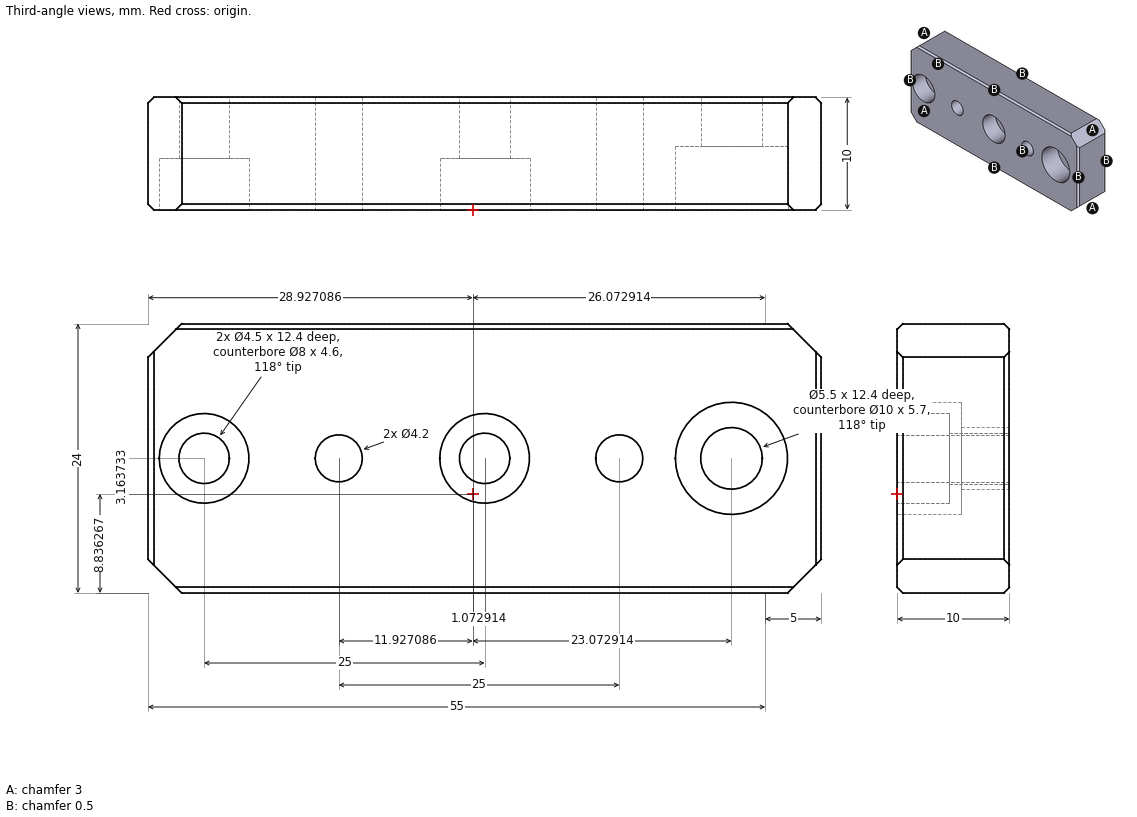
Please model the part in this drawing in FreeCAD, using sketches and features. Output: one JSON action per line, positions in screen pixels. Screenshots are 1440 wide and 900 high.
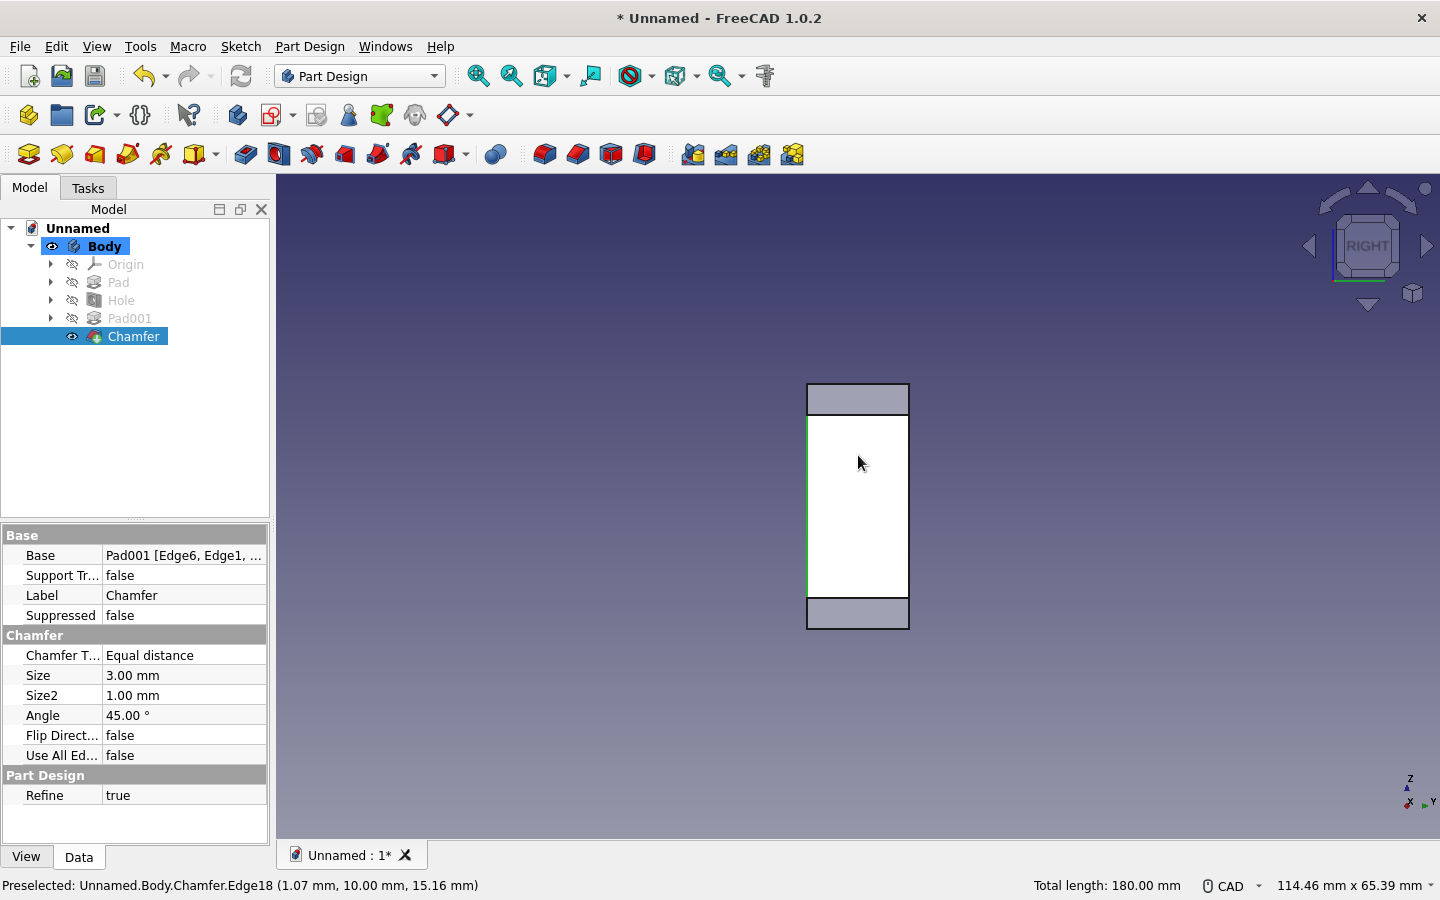
{"action": "left_click", "coordinate": [909, 505], "text": "ctrl"}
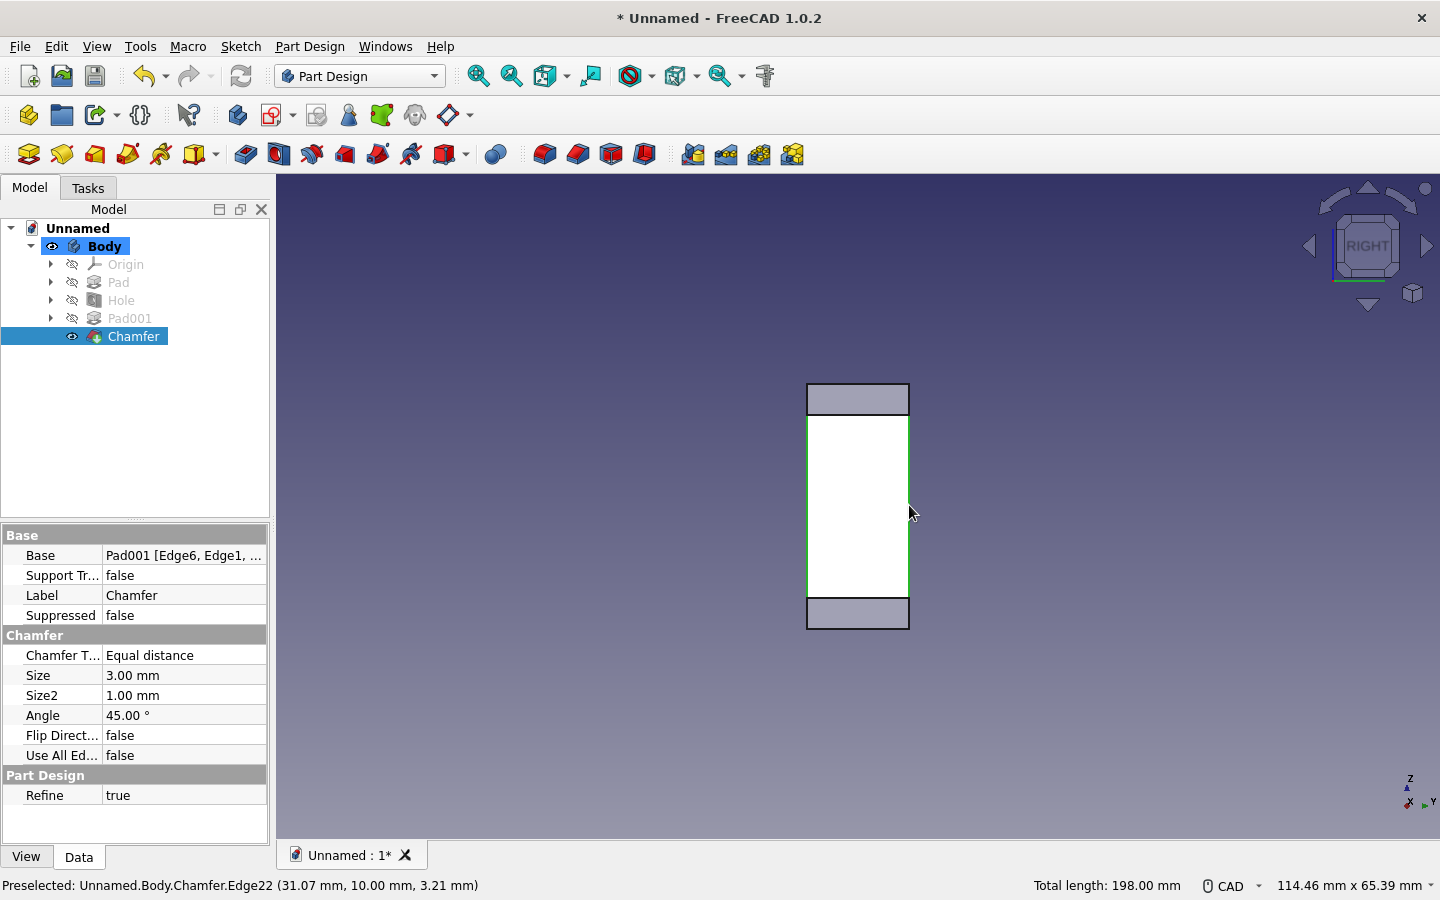
{"action": "key", "text": "5"}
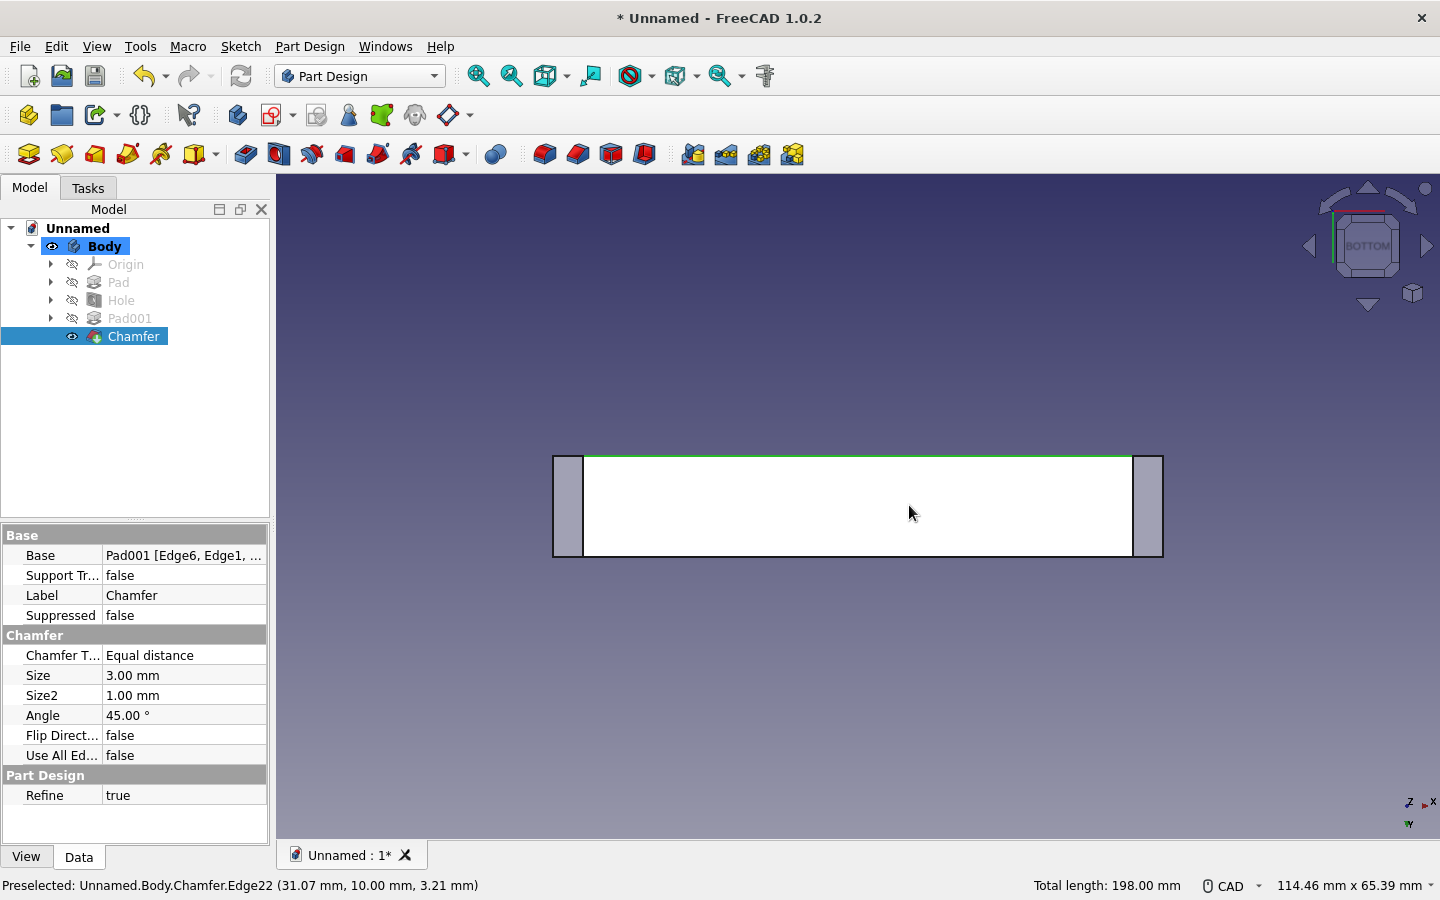
{"action": "key", "text": "4"}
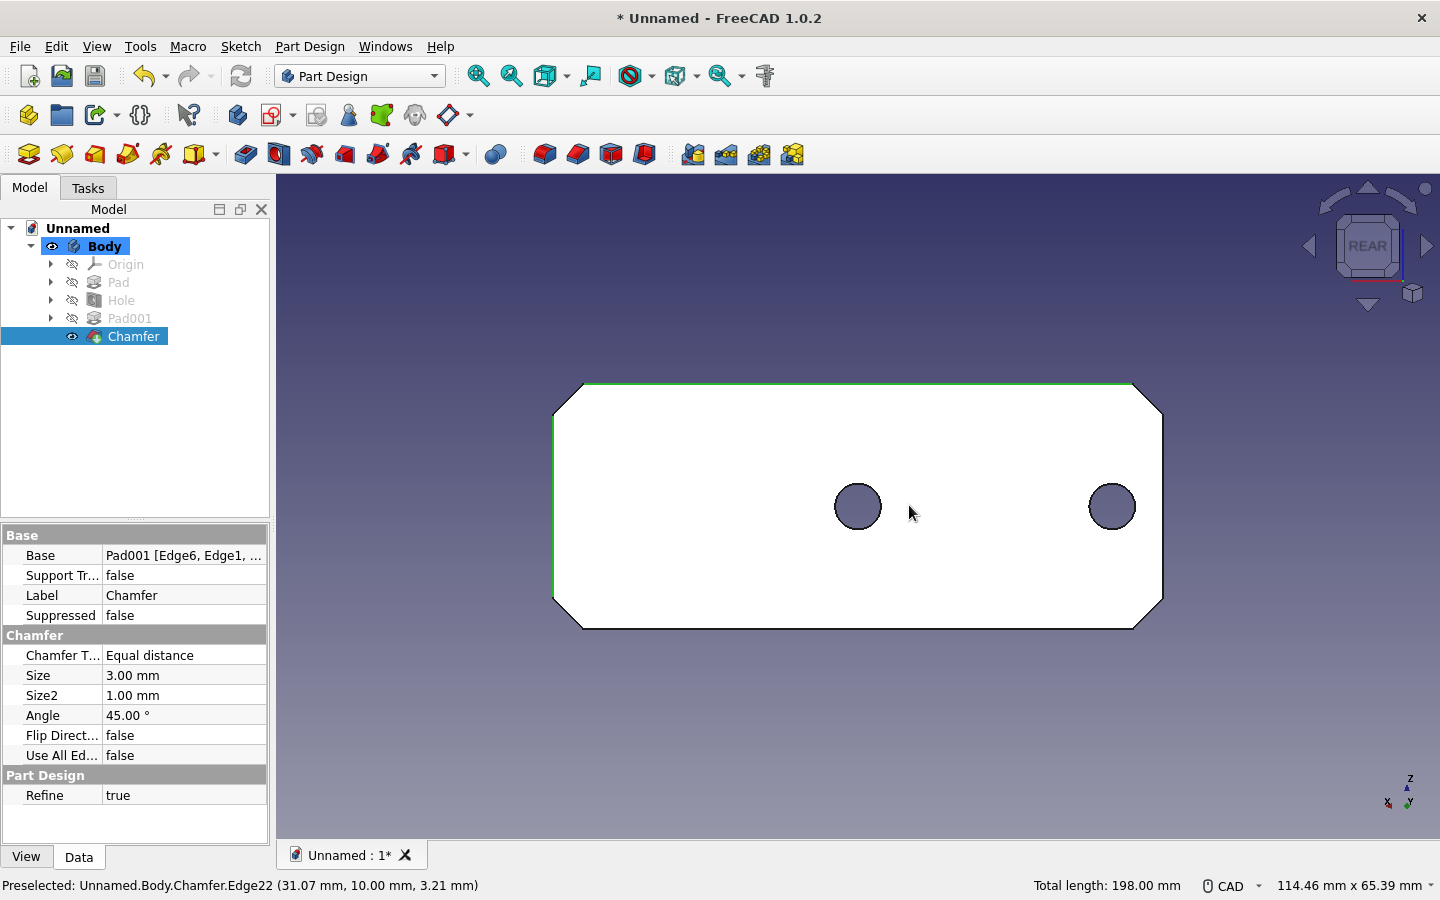
{"action": "left_click", "coordinate": [858, 628], "text": "ctrl"}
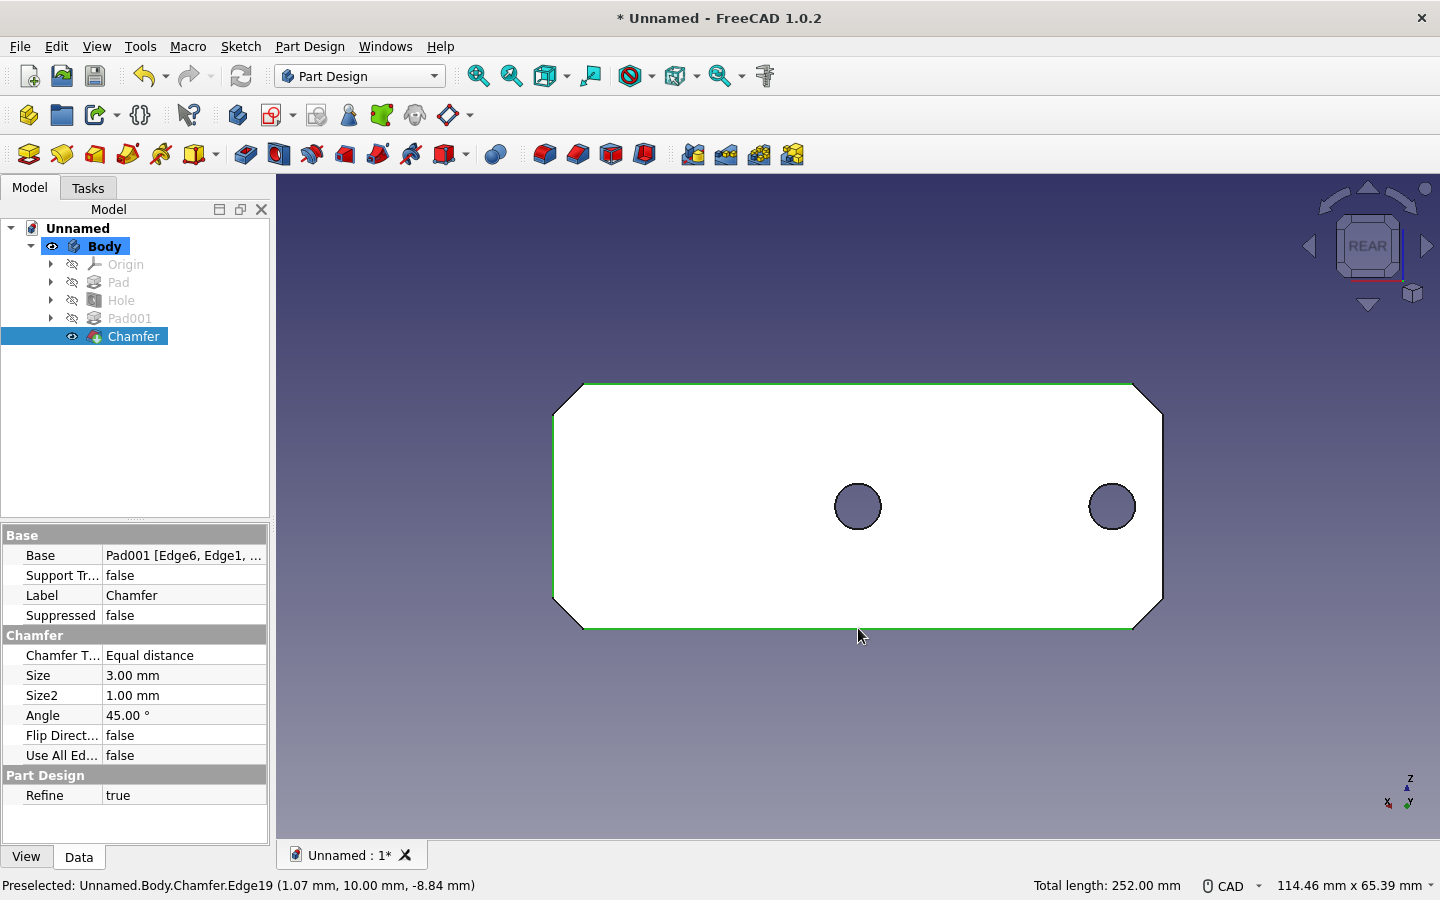
{"action": "left_click", "coordinate": [1163, 506], "text": "ctrl"}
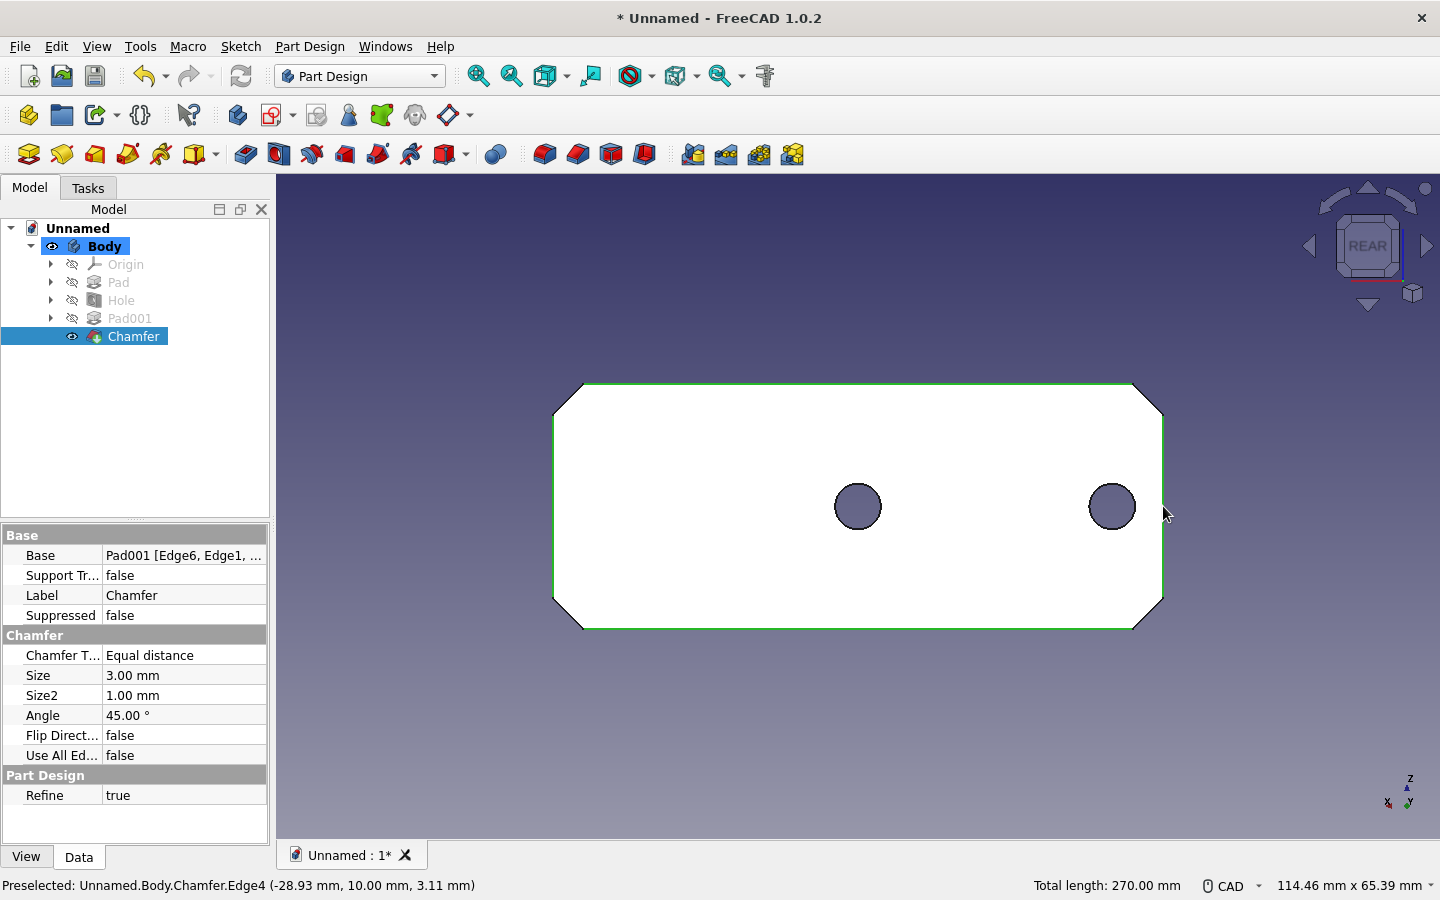
{"action": "key", "text": "6"}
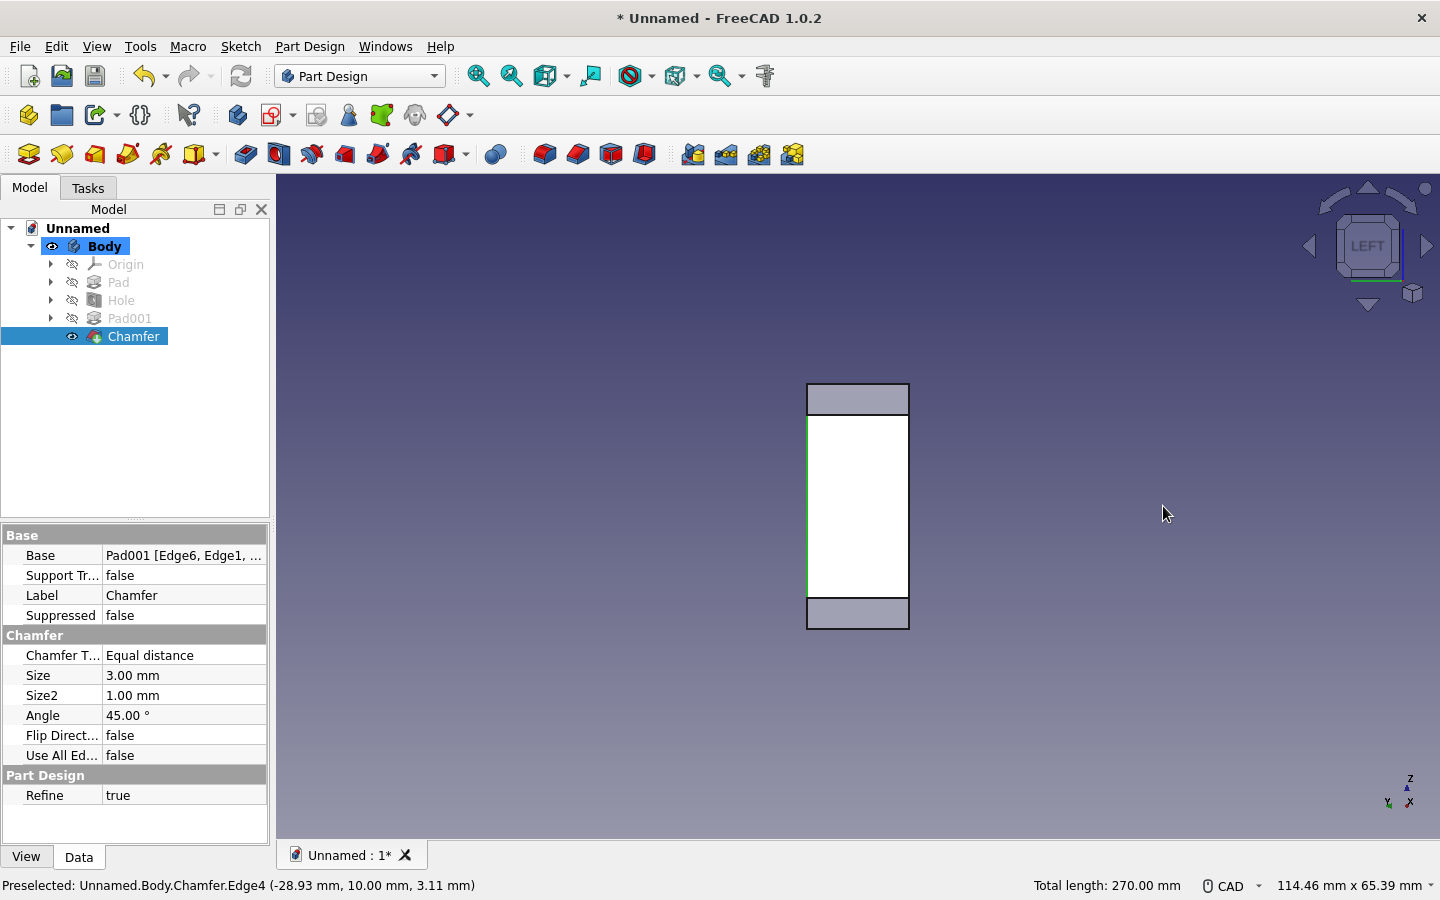
{"action": "key", "text": "v f"}